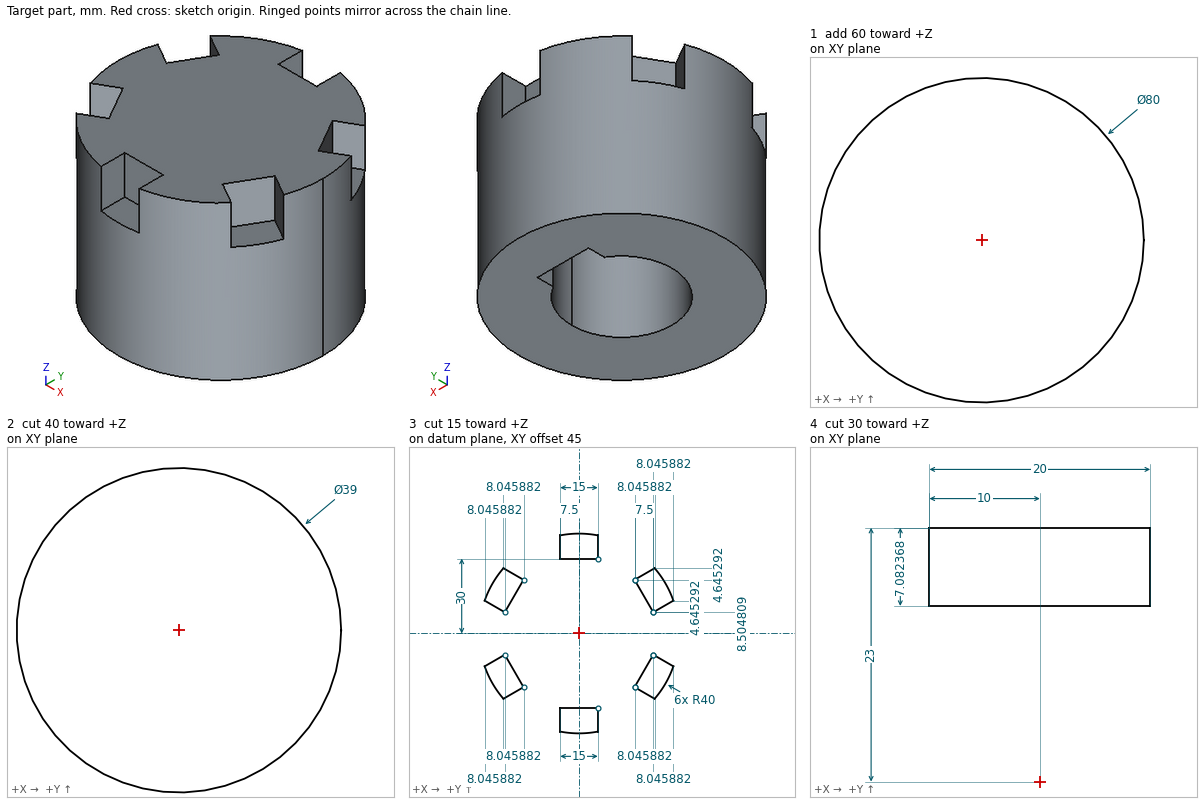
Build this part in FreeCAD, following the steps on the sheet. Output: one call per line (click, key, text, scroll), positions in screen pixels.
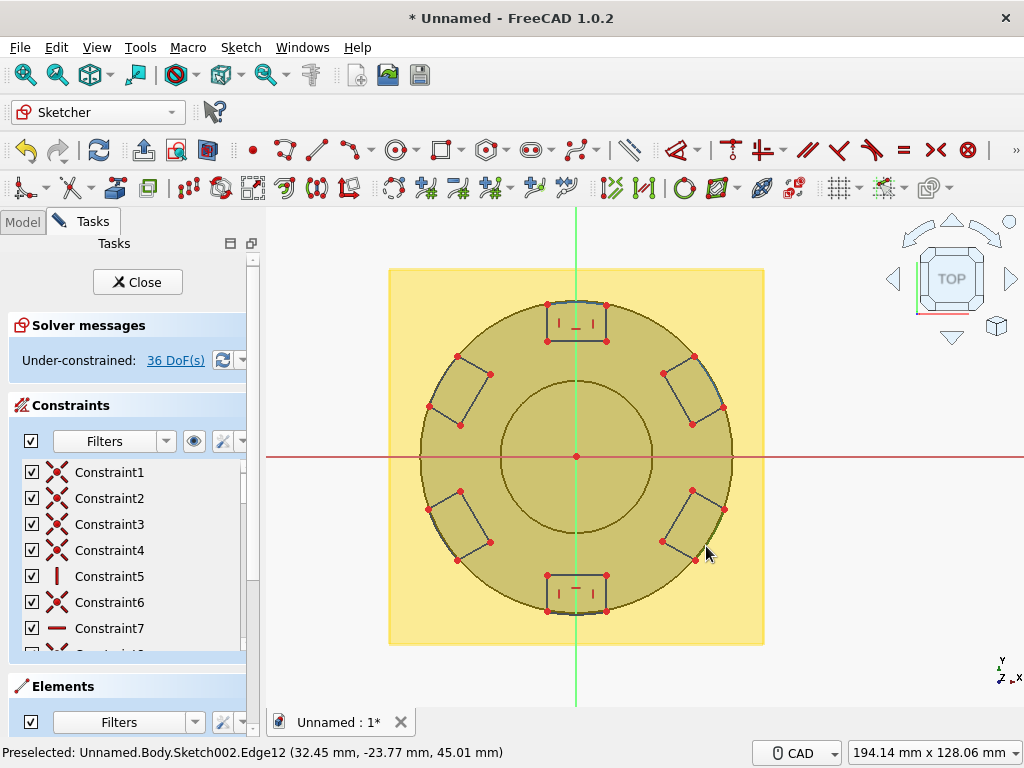
click(565, 614)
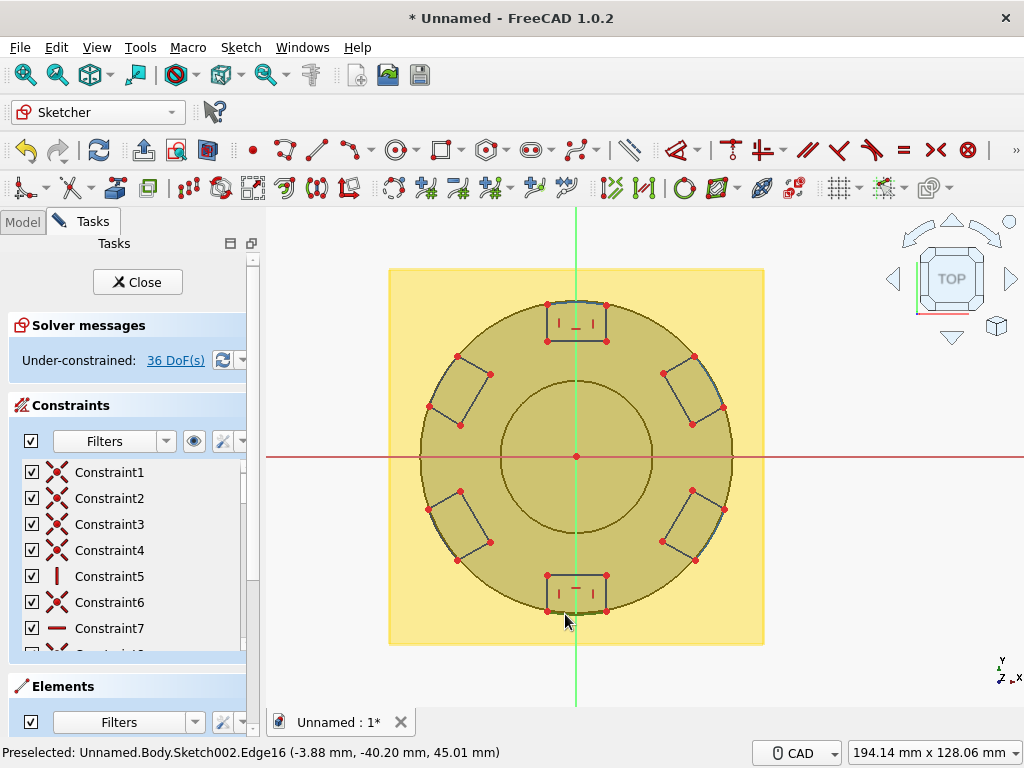
click(435, 526)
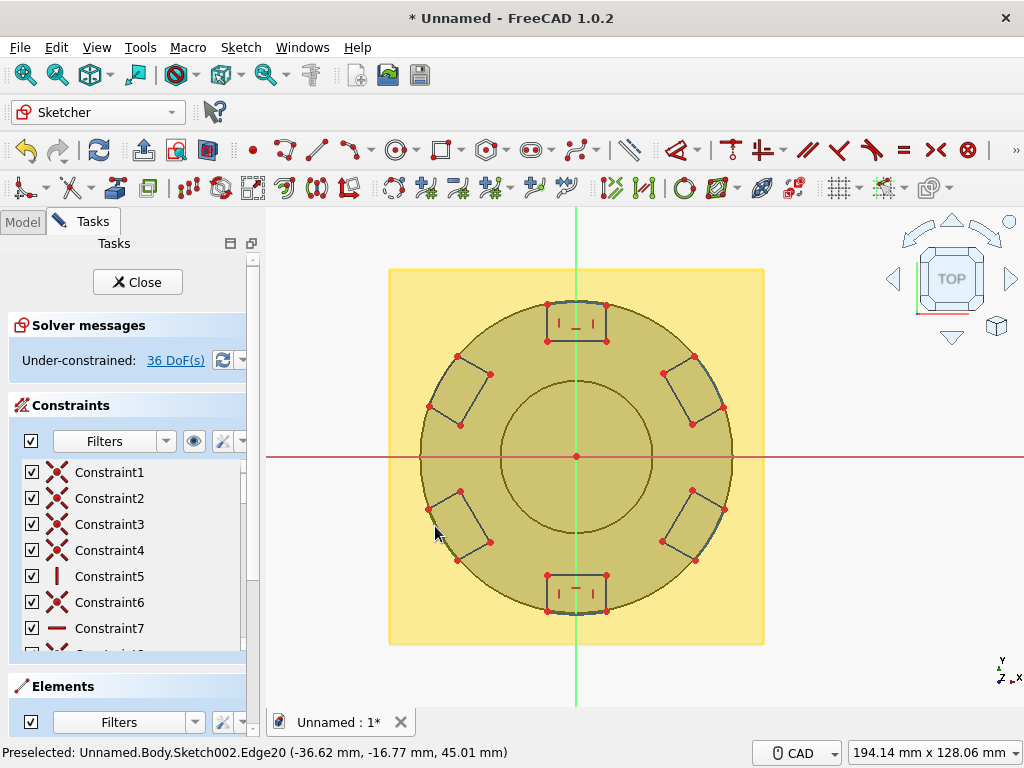
click(447, 370)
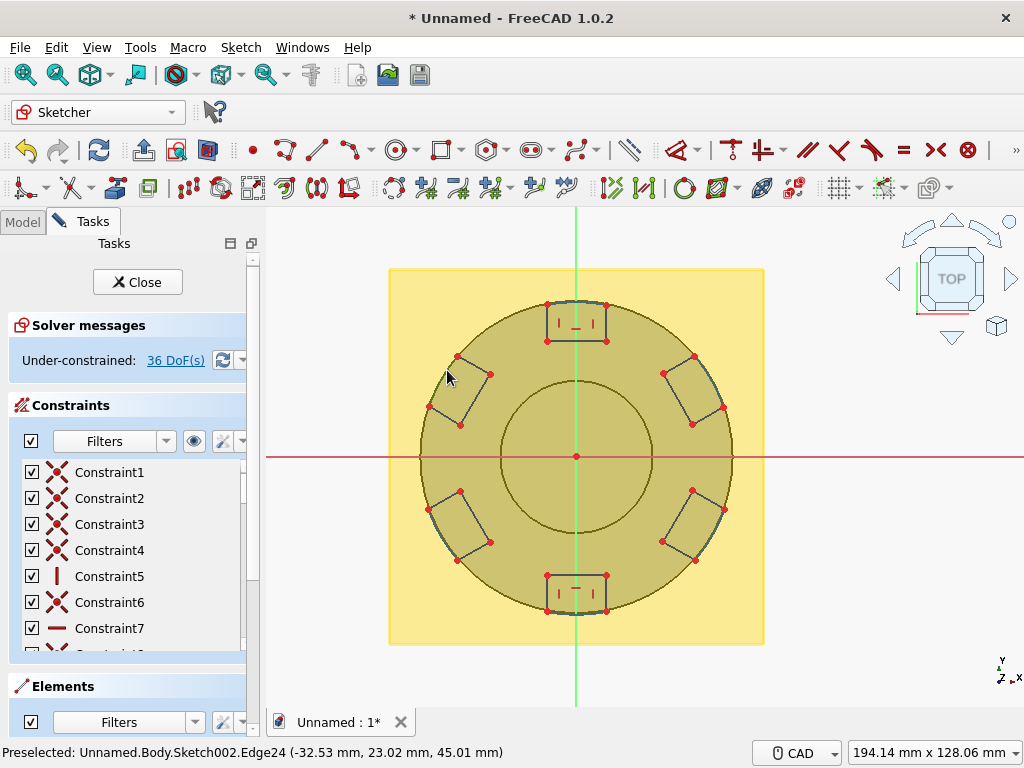
click(904, 150)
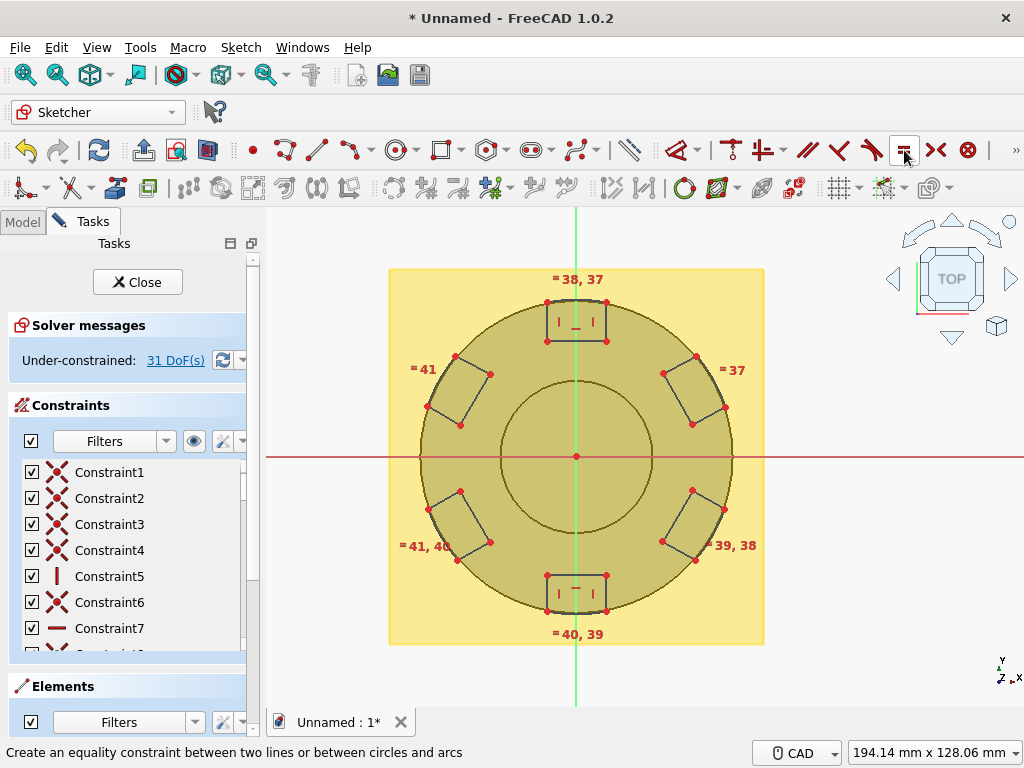
click(692, 425)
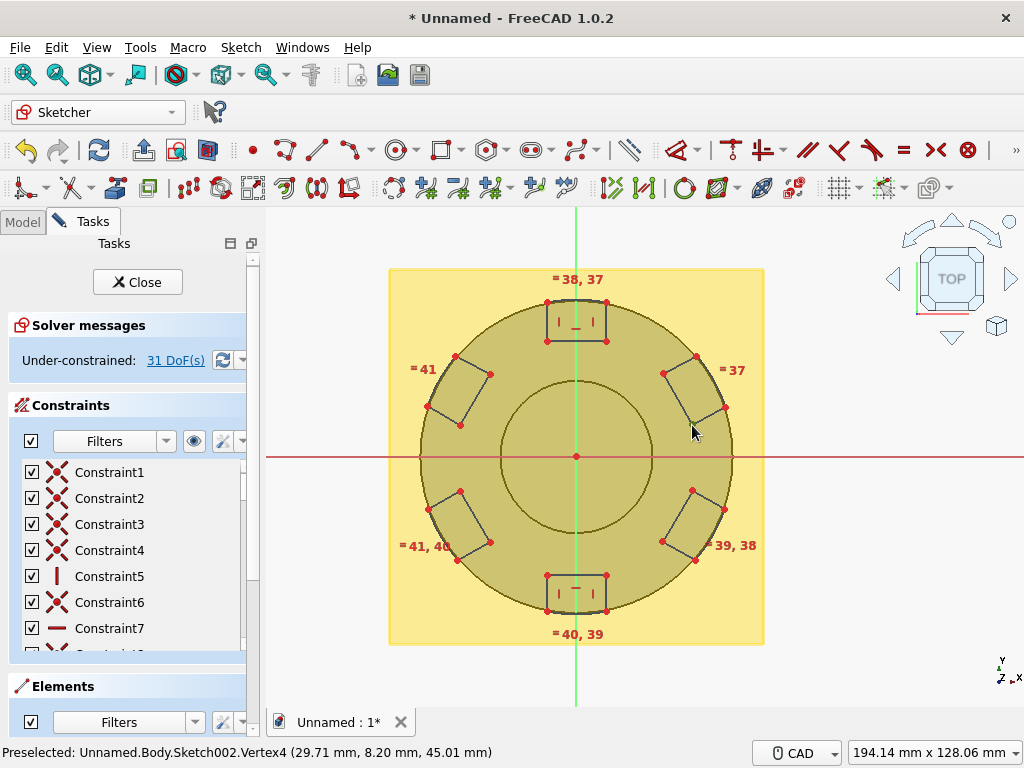
click(693, 491)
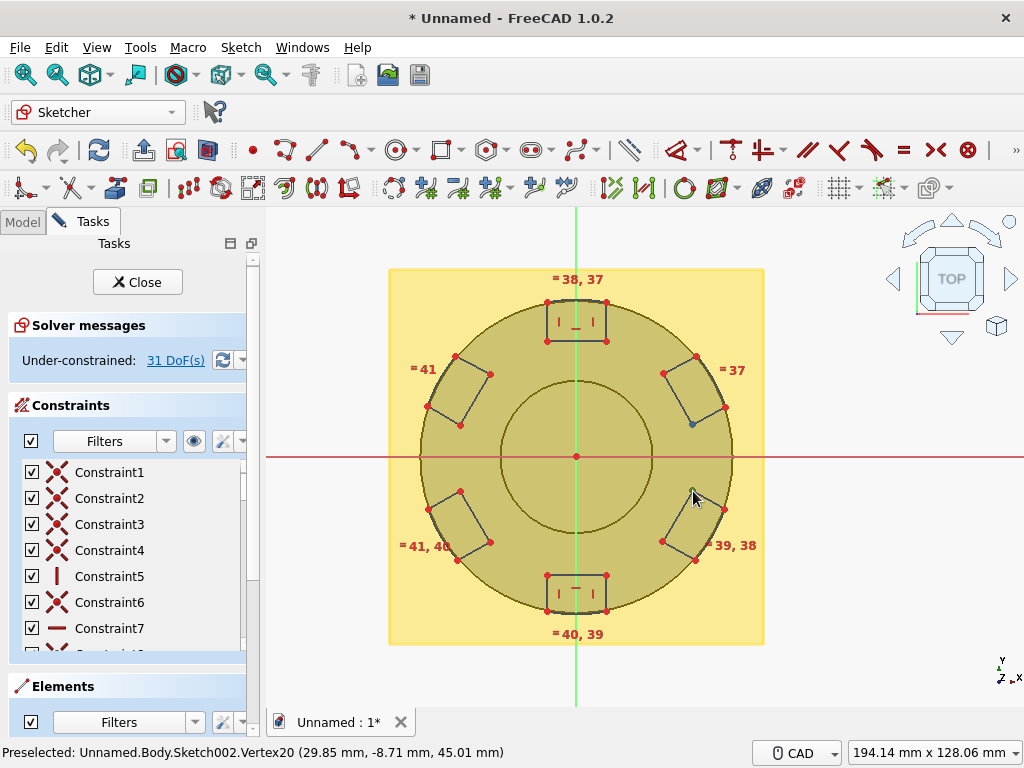
click(334, 457)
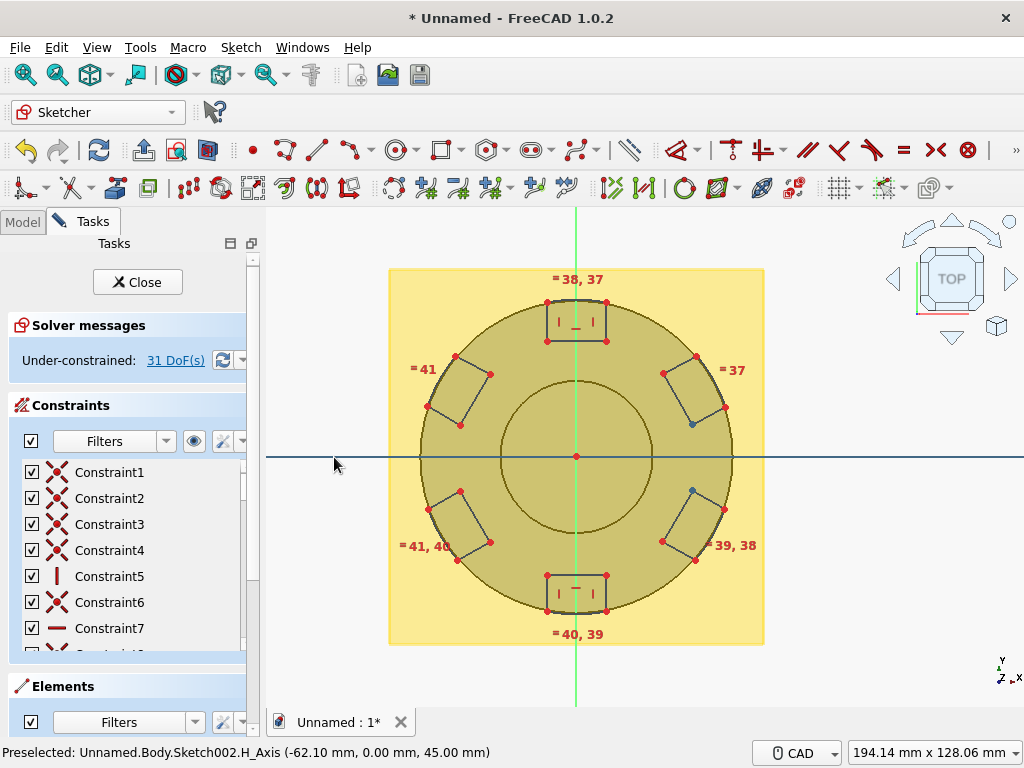
click(936, 150)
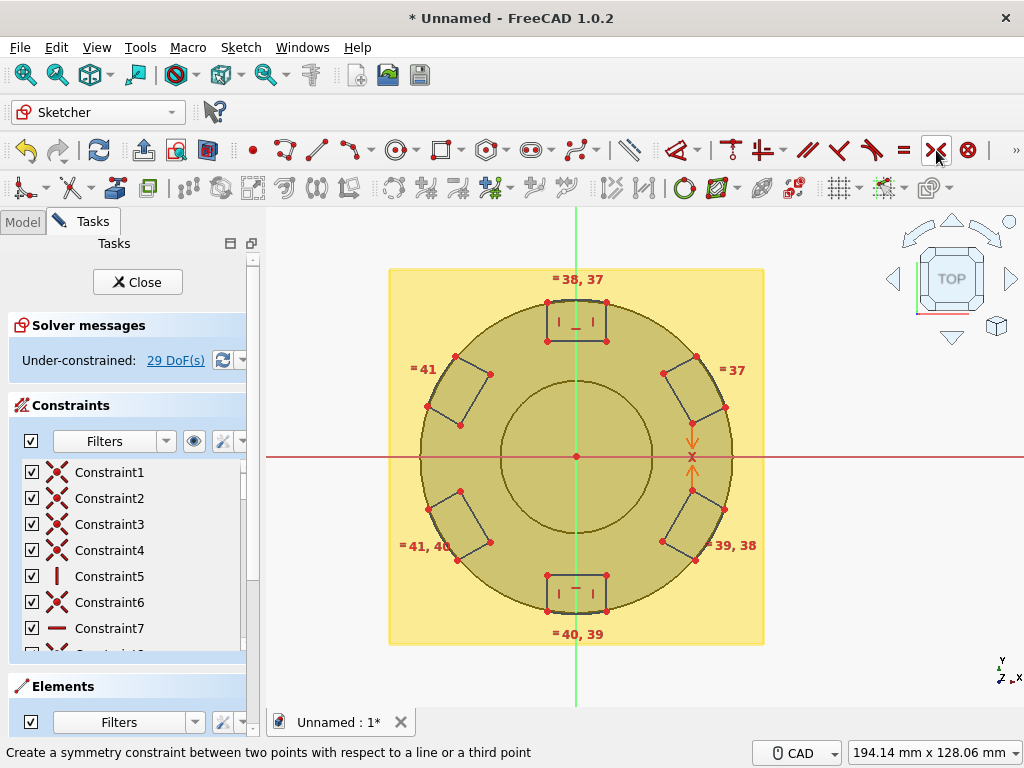
click(663, 374)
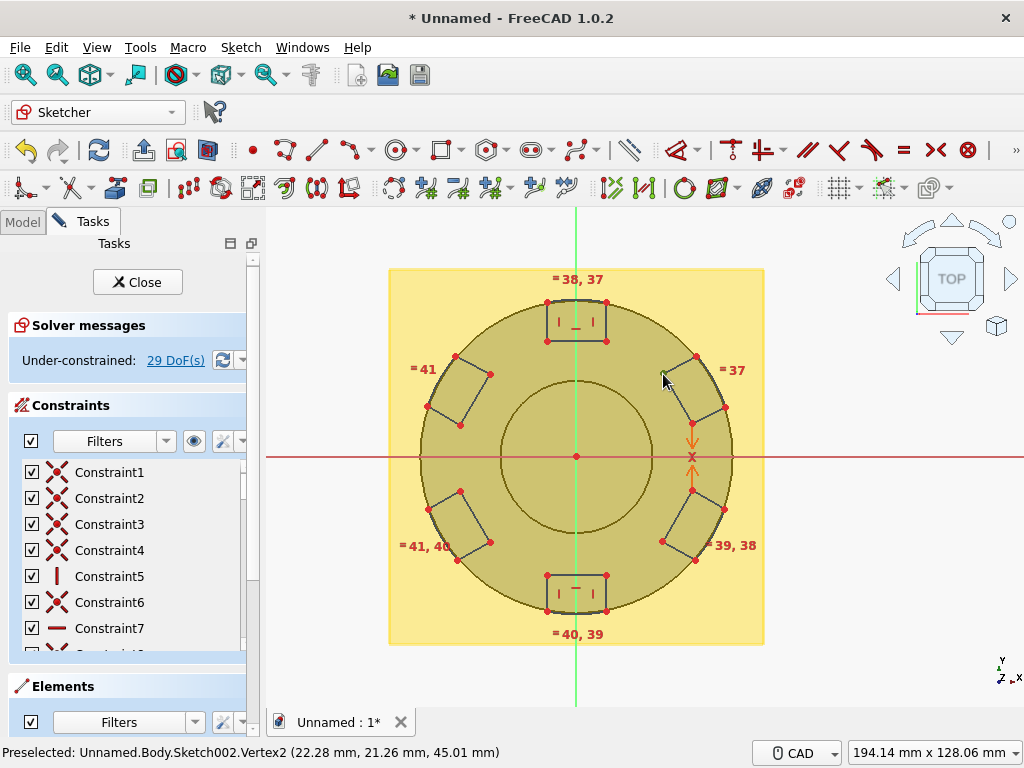
click(663, 542)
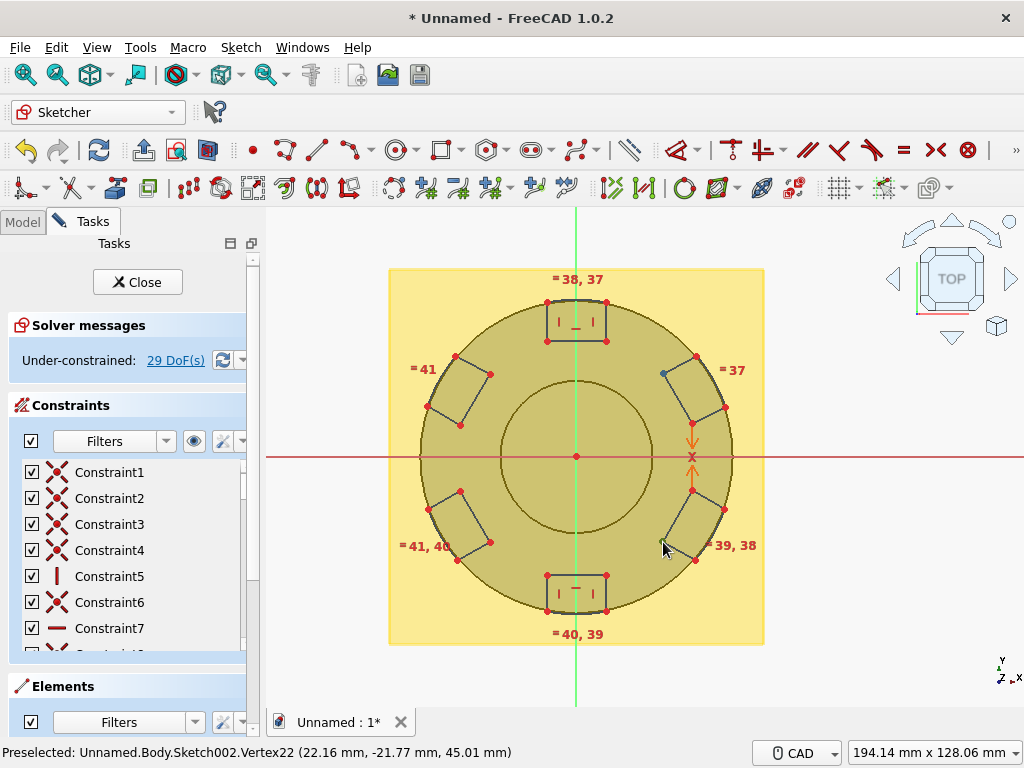
click(334, 457)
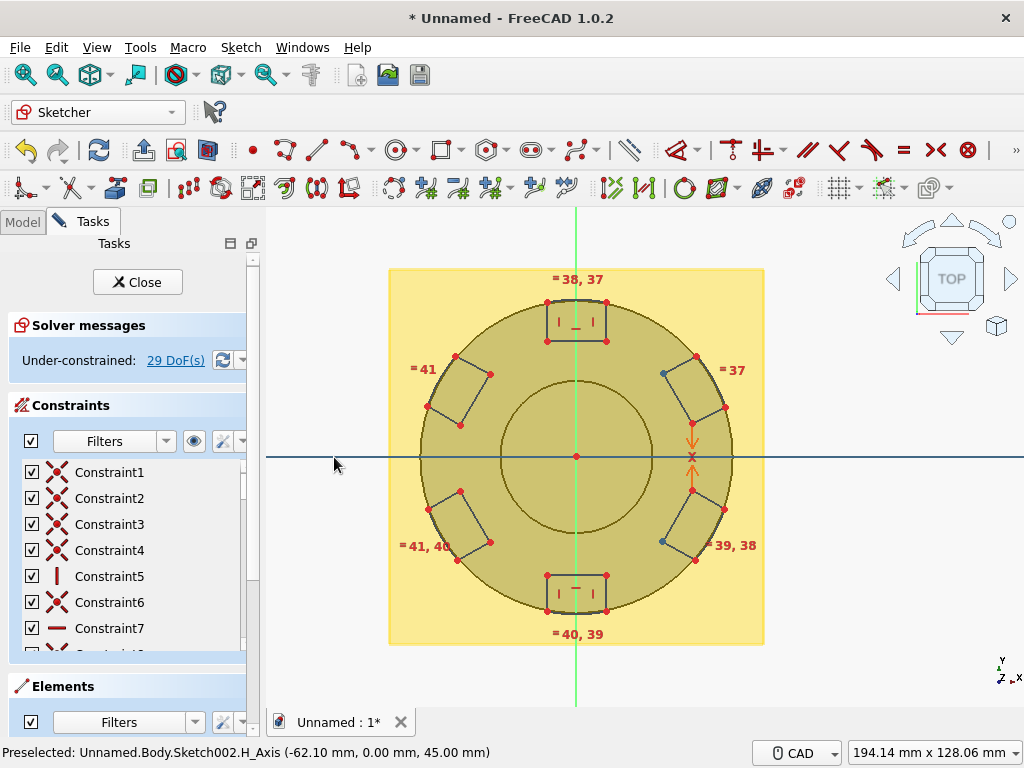
click(936, 150)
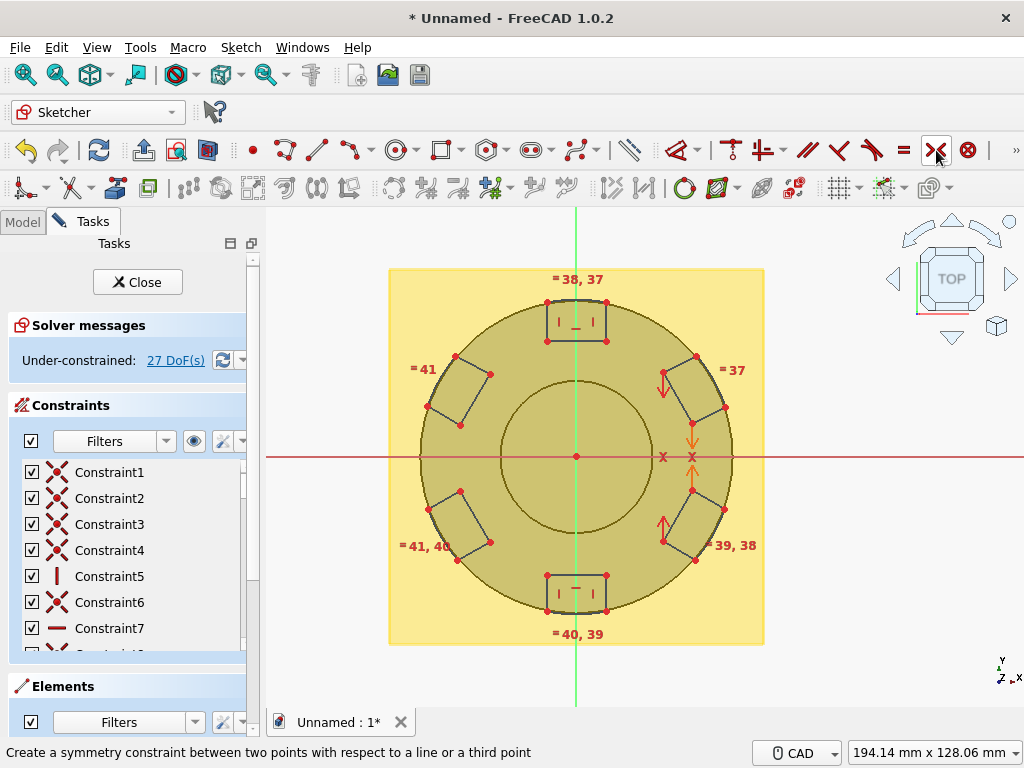
click(606, 341)